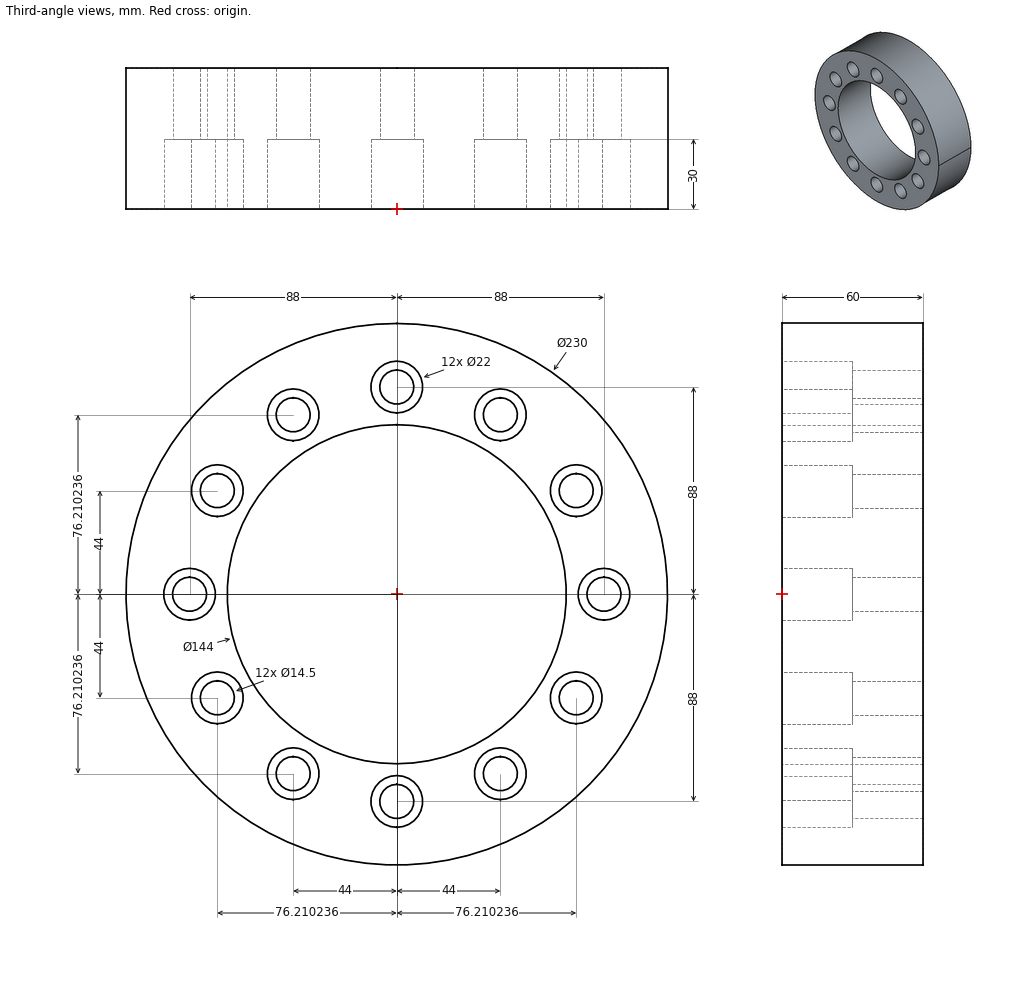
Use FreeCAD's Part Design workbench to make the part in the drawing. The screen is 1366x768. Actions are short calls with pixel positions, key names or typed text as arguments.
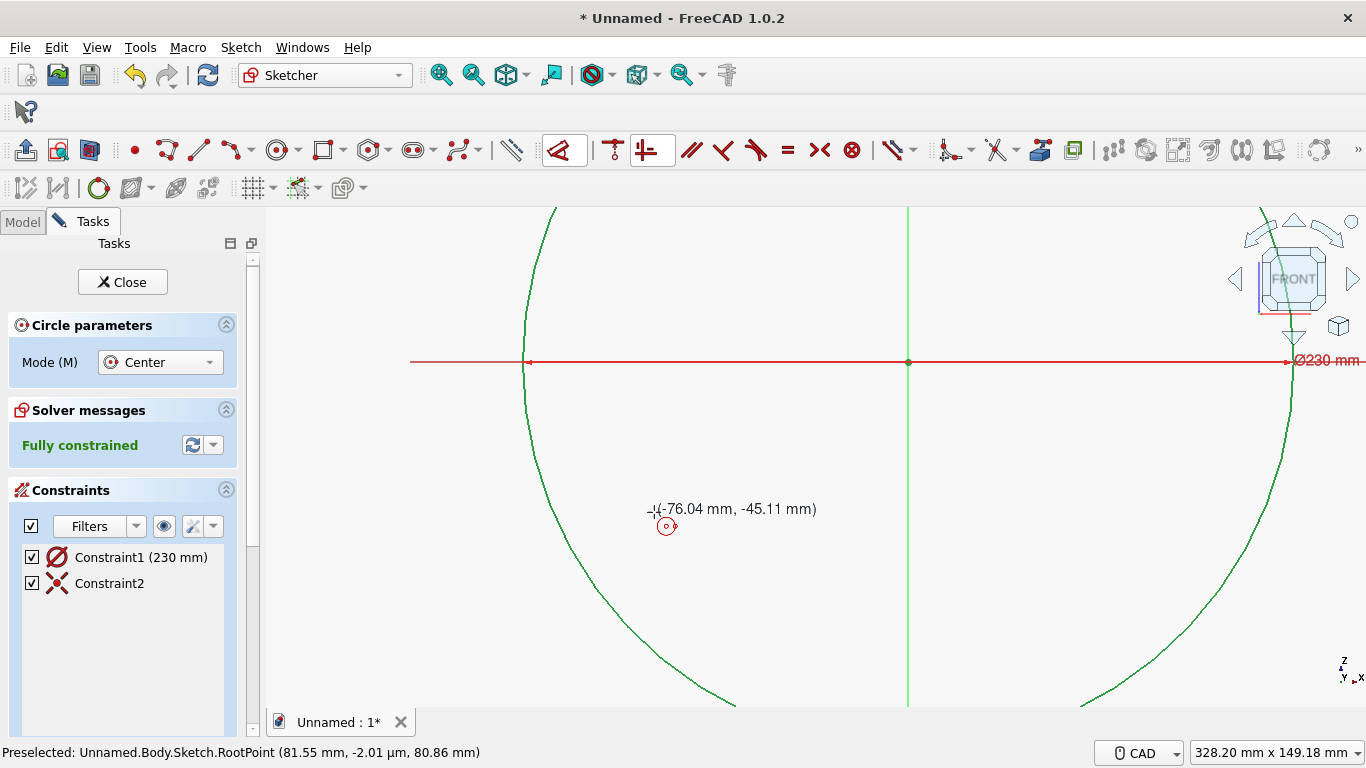
click(653, 510)
move(670, 493)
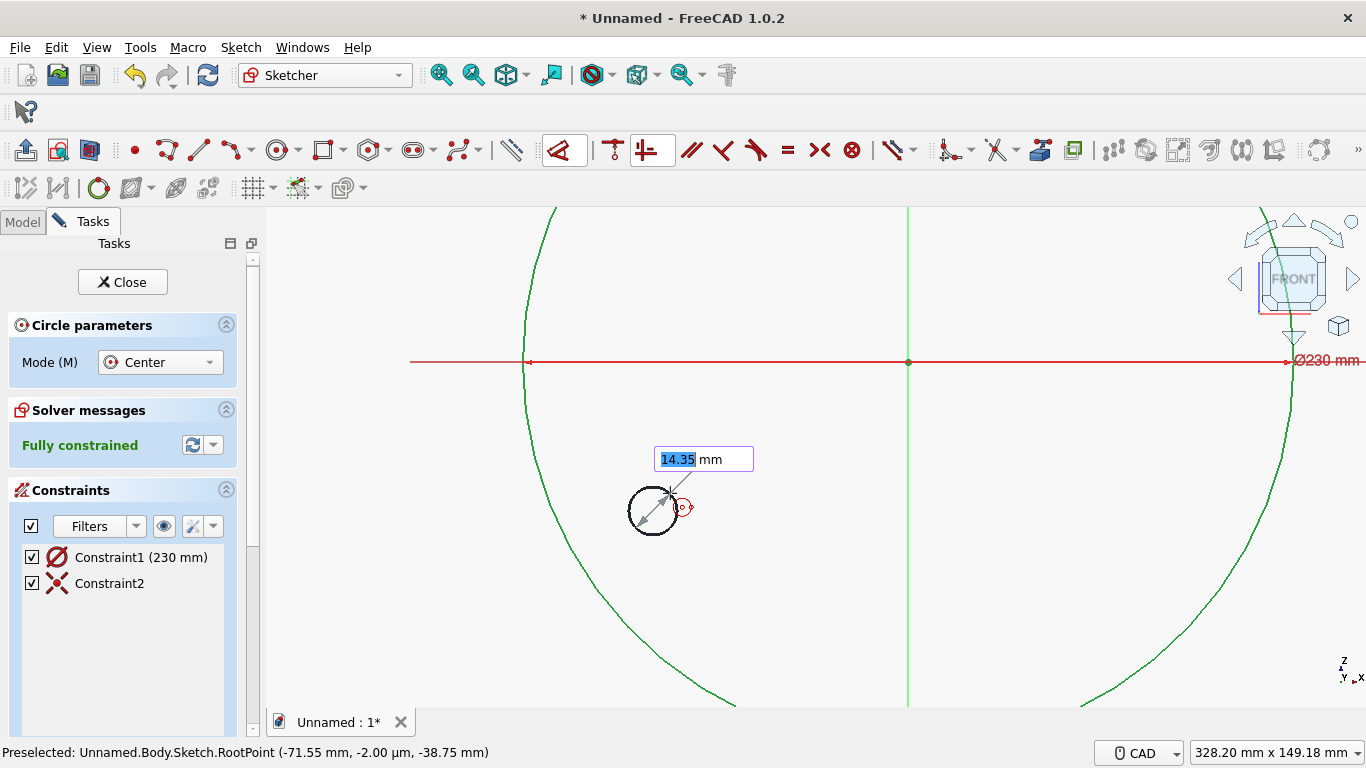
text(14.5)
key(Return)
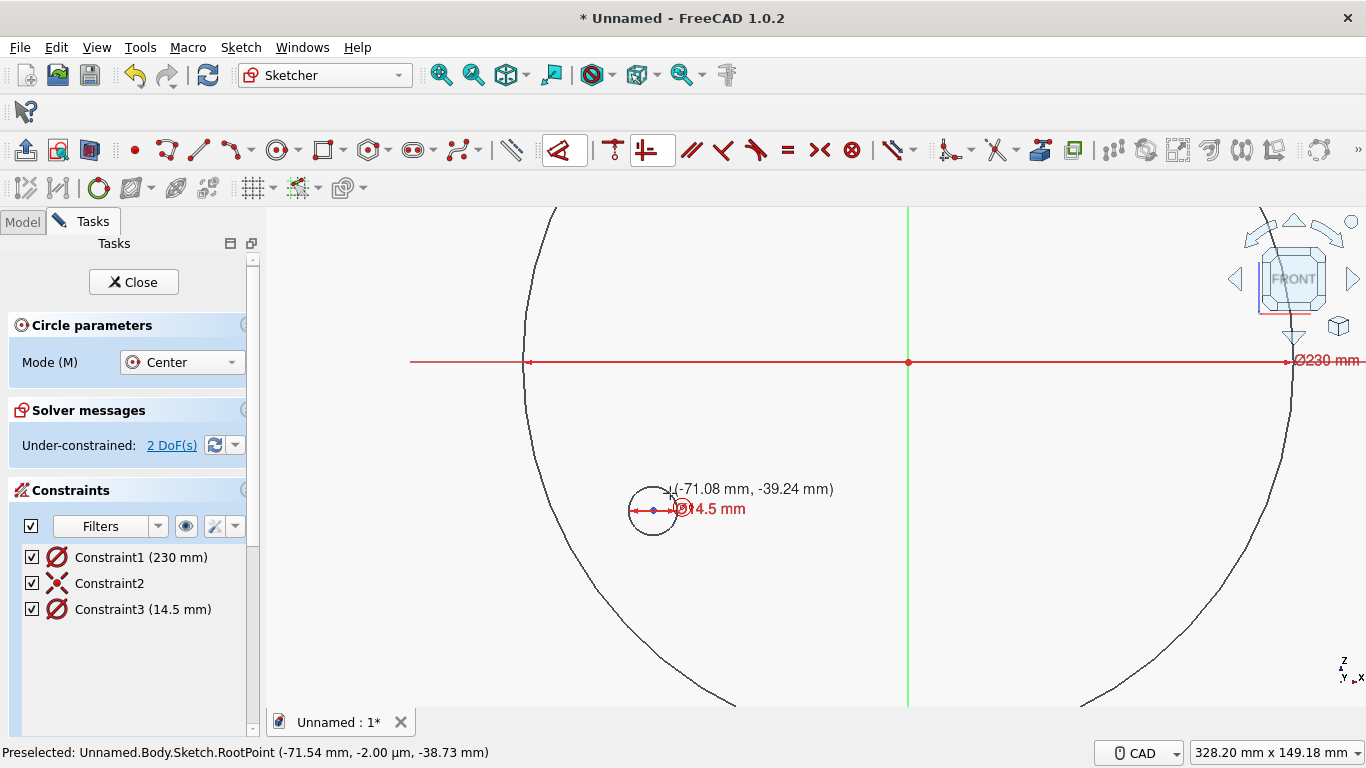
click(761, 618)
move(778, 601)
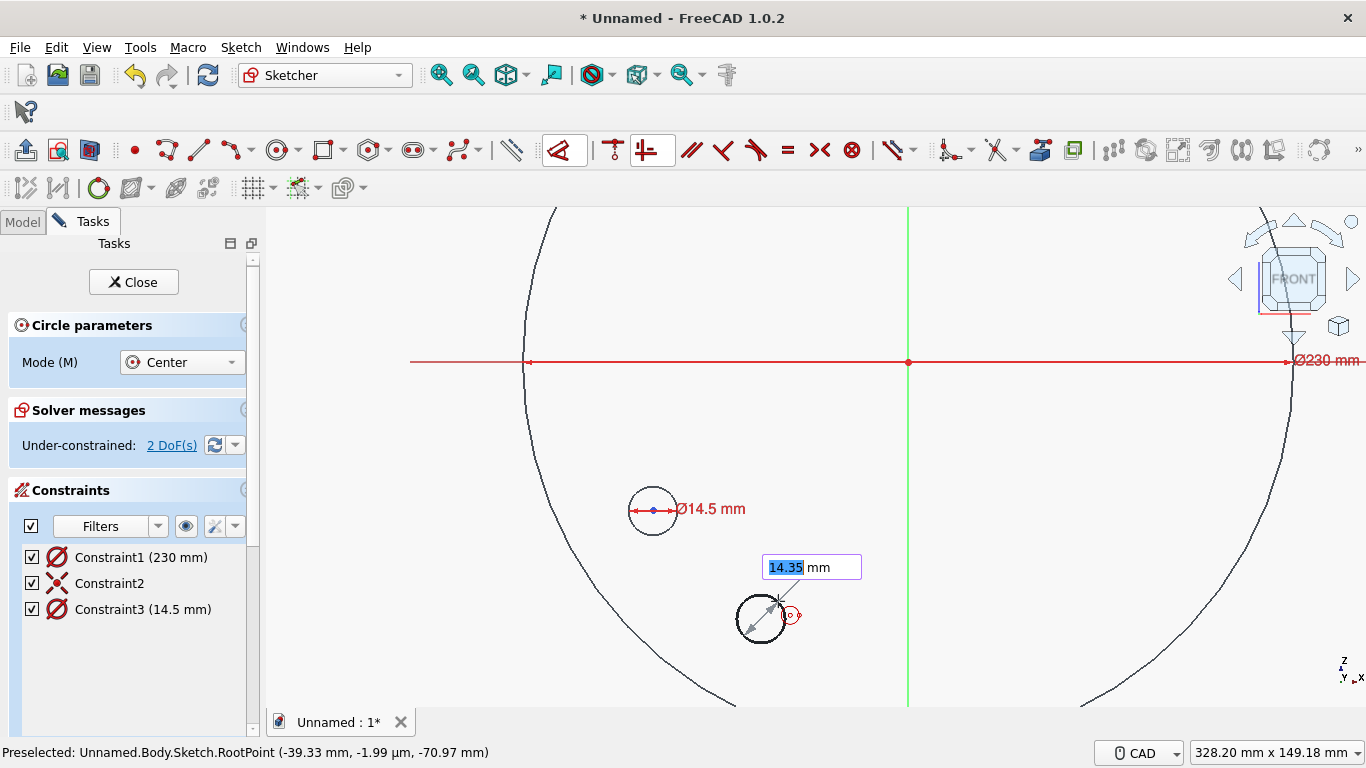
text(14.5)
key(Return)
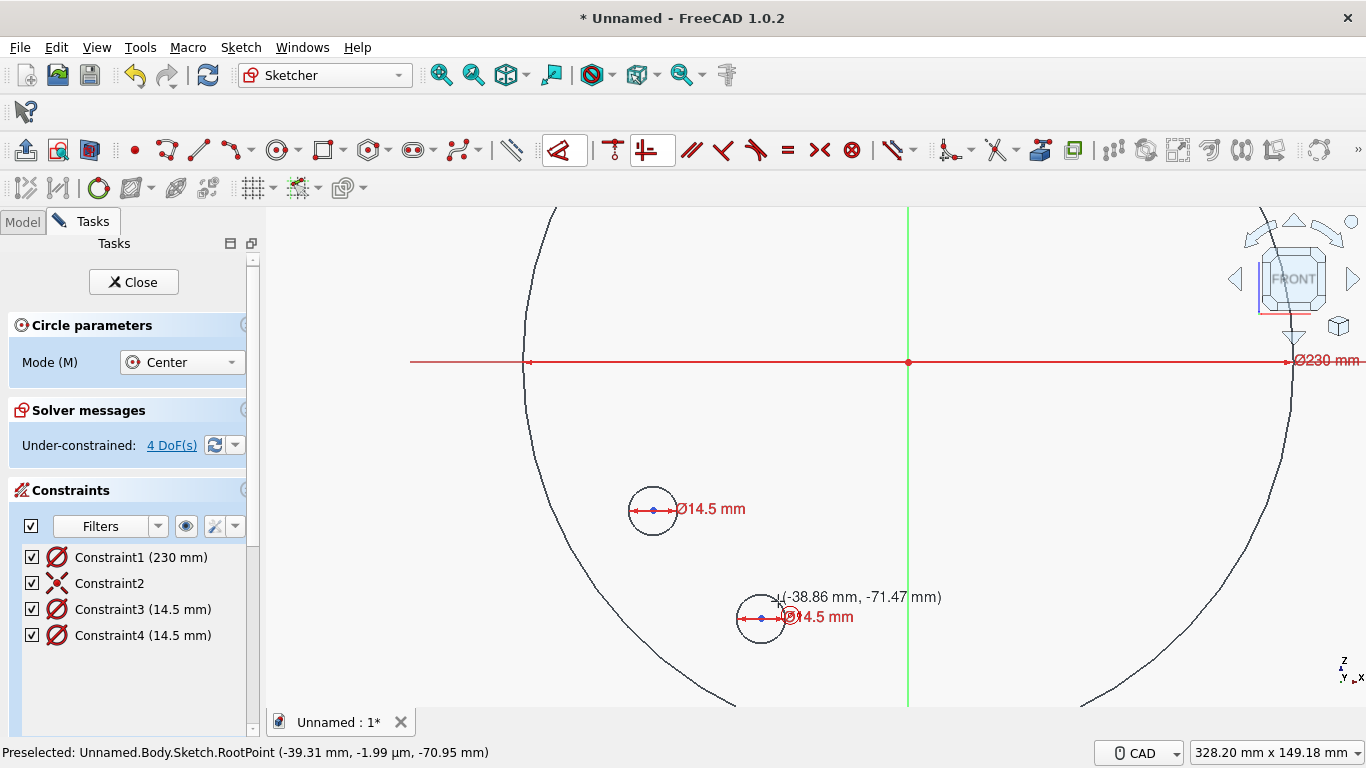
click(908, 657)
move(925, 640)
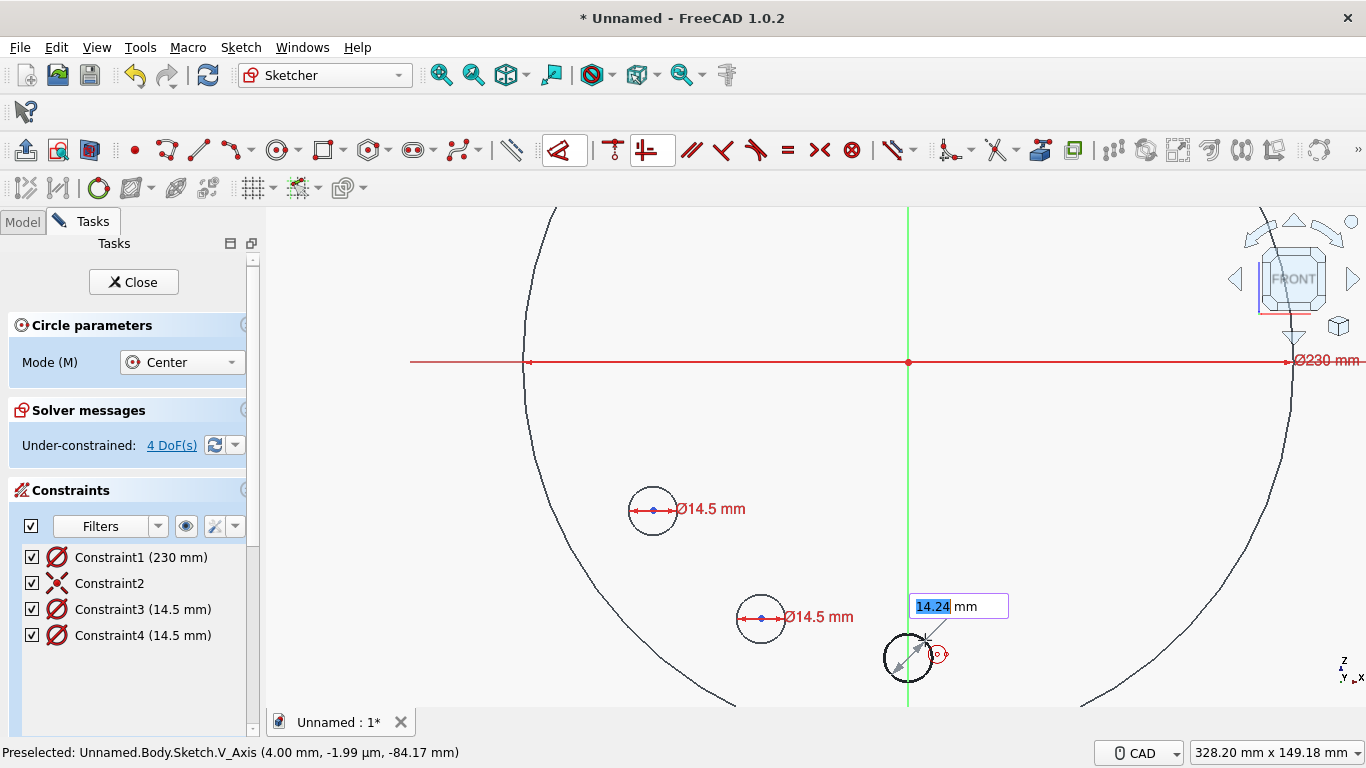
text(14.5)
key(Return)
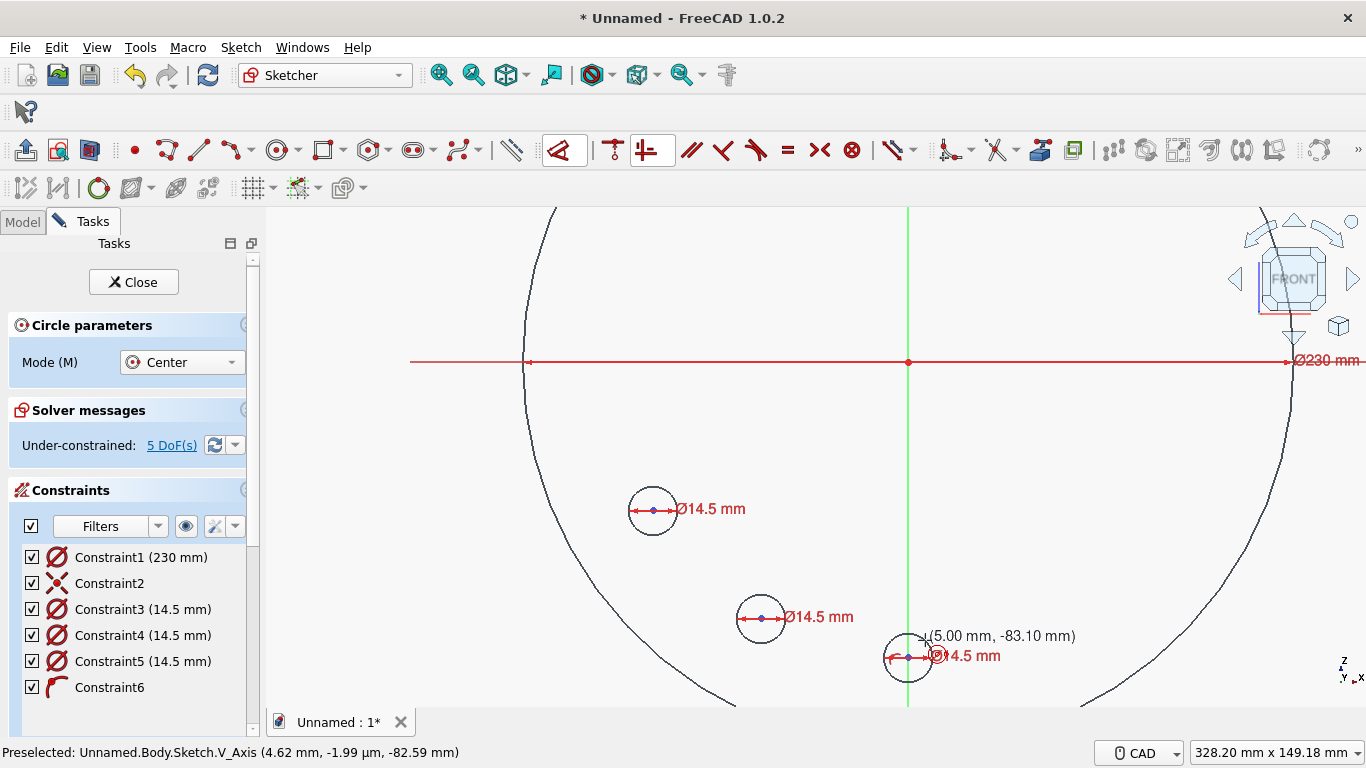
click(613, 362)
move(630, 345)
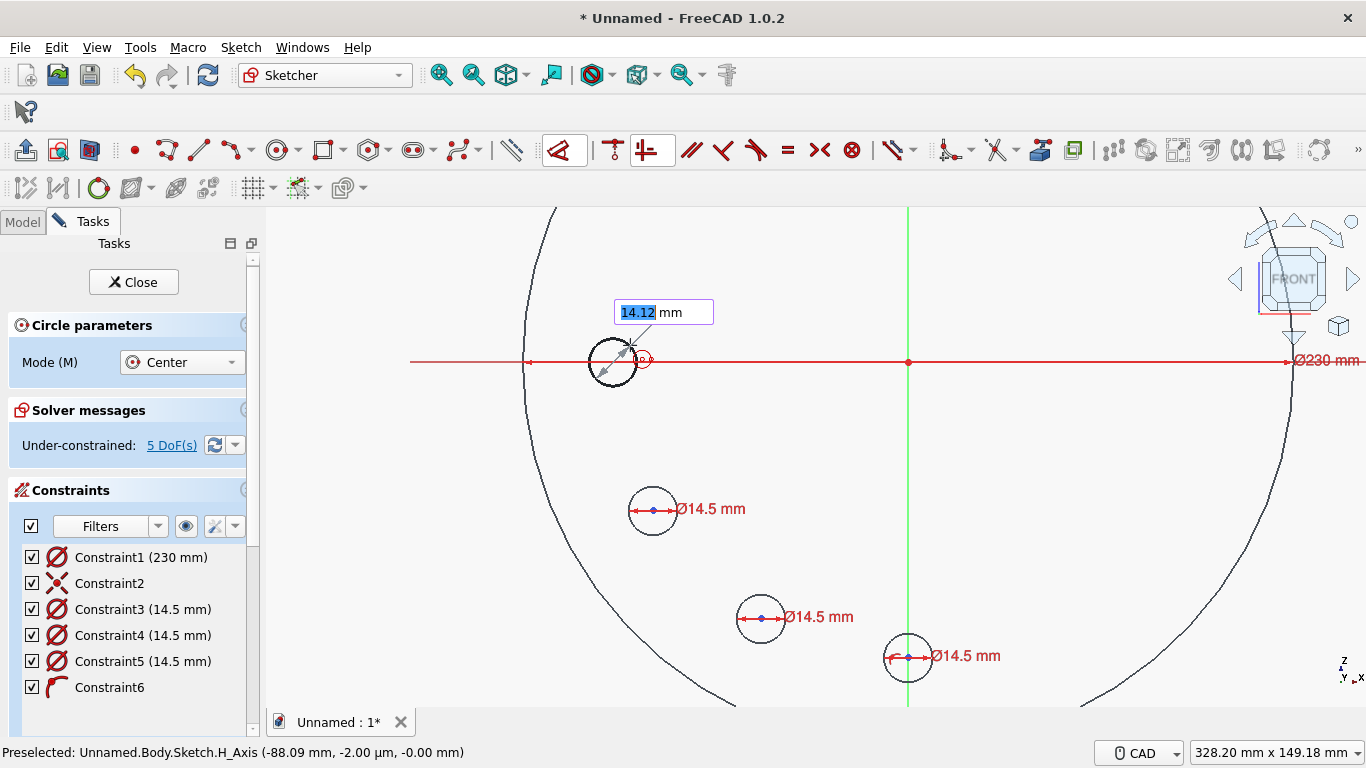
text(14.5)
key(Return)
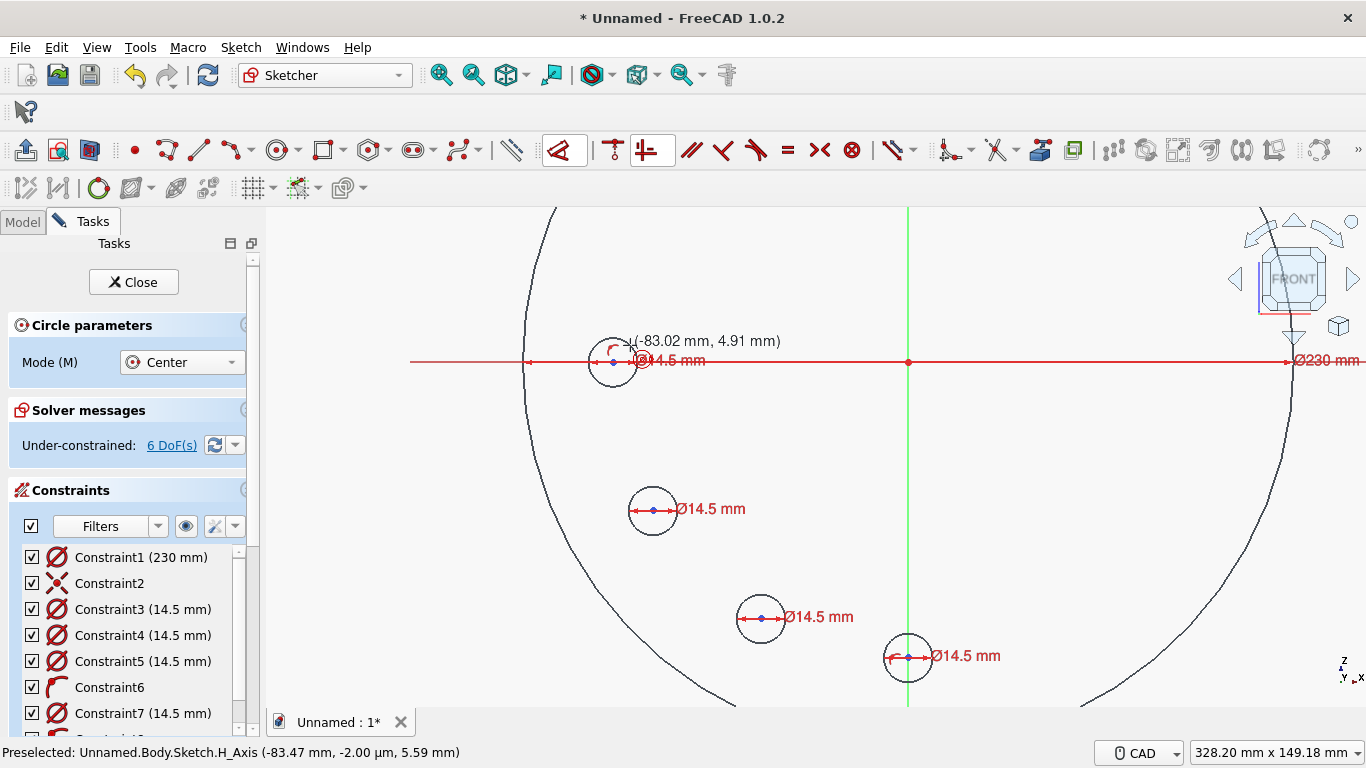
scroll(654, 512, down, 5)